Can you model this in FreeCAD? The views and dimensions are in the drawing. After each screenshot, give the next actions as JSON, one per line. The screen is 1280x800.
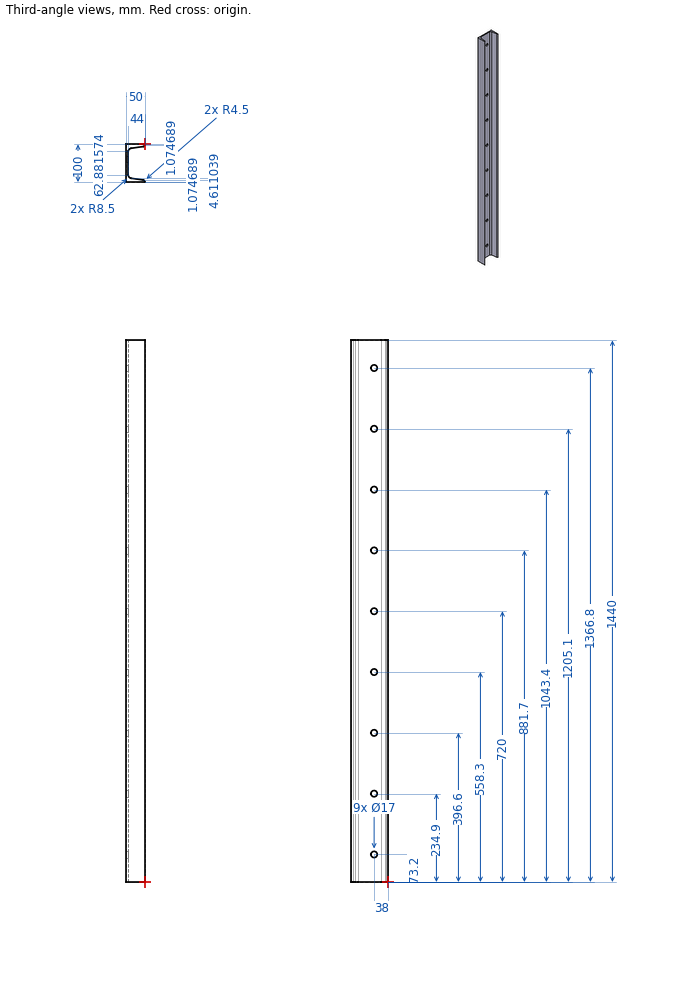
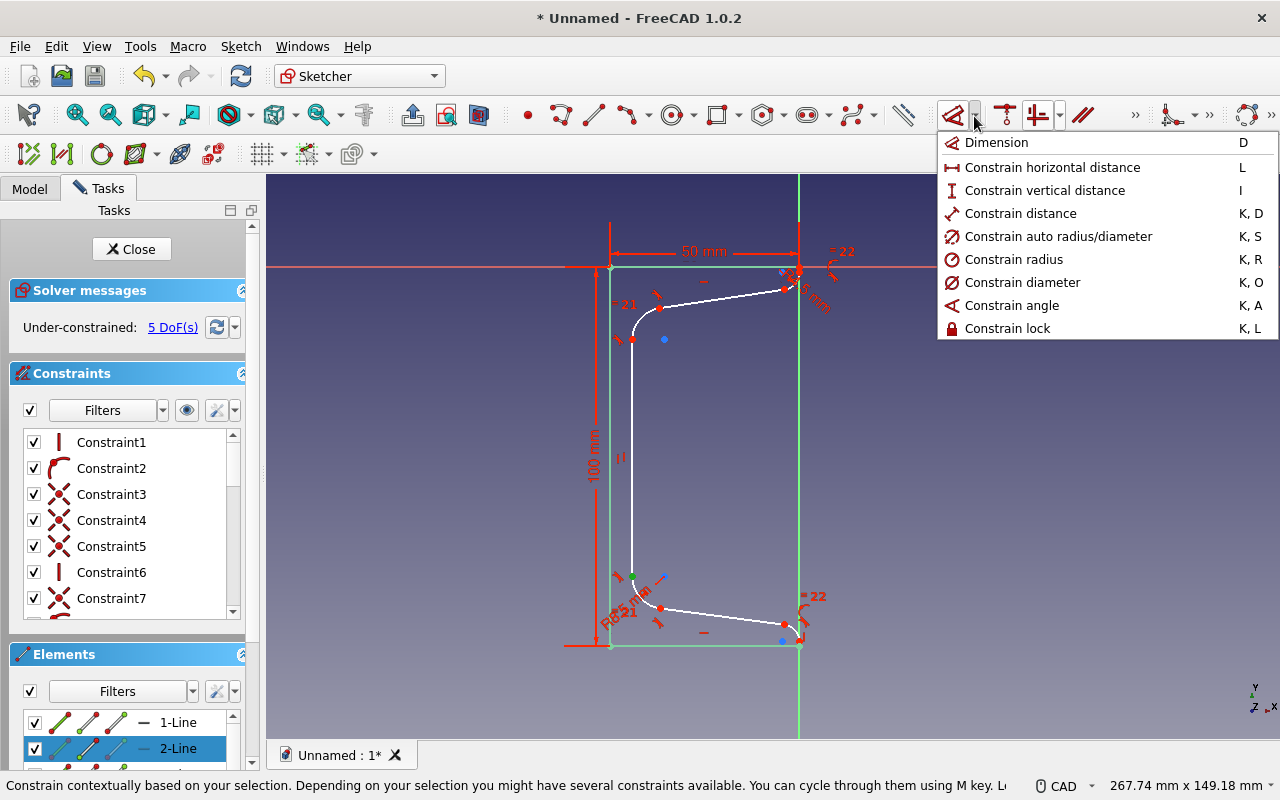
{"action": "left_click", "coordinate": [1108, 168]}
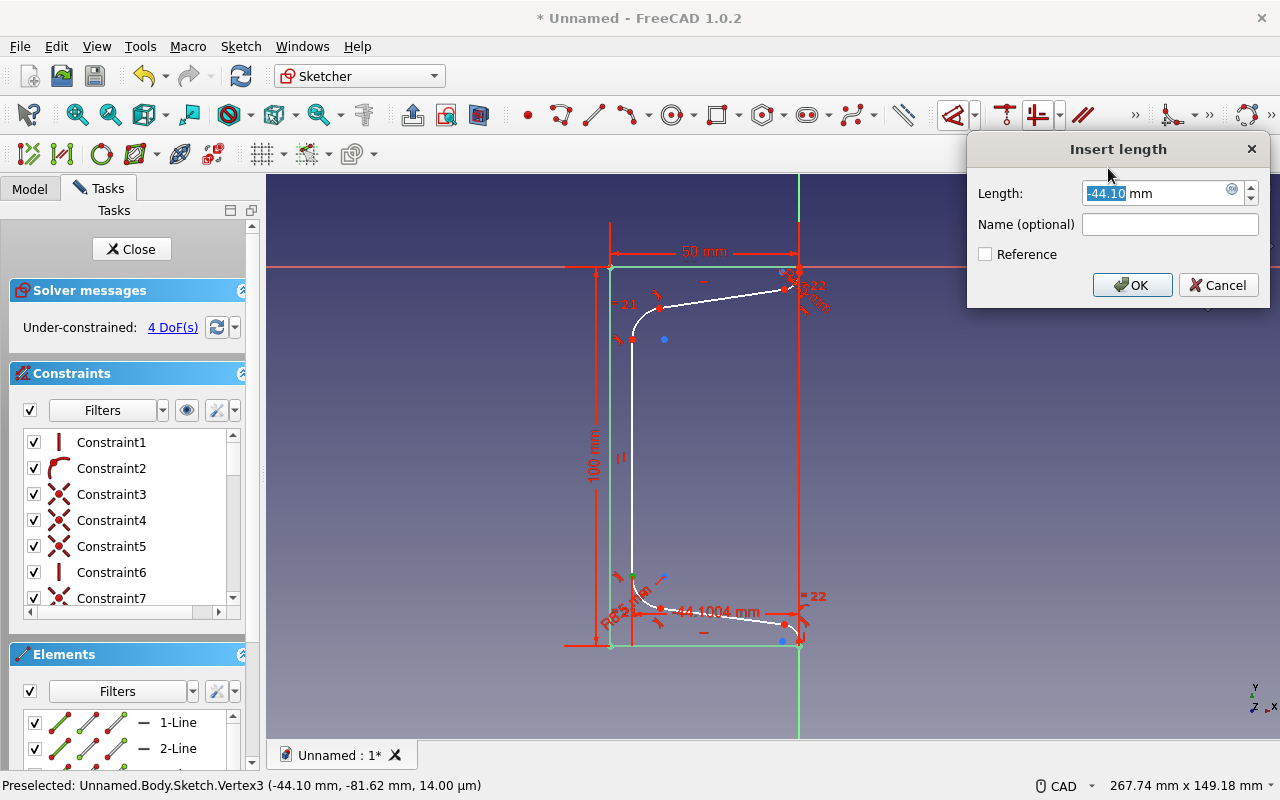
{"action": "type", "text": "-44"}
{"action": "key", "text": "Return"}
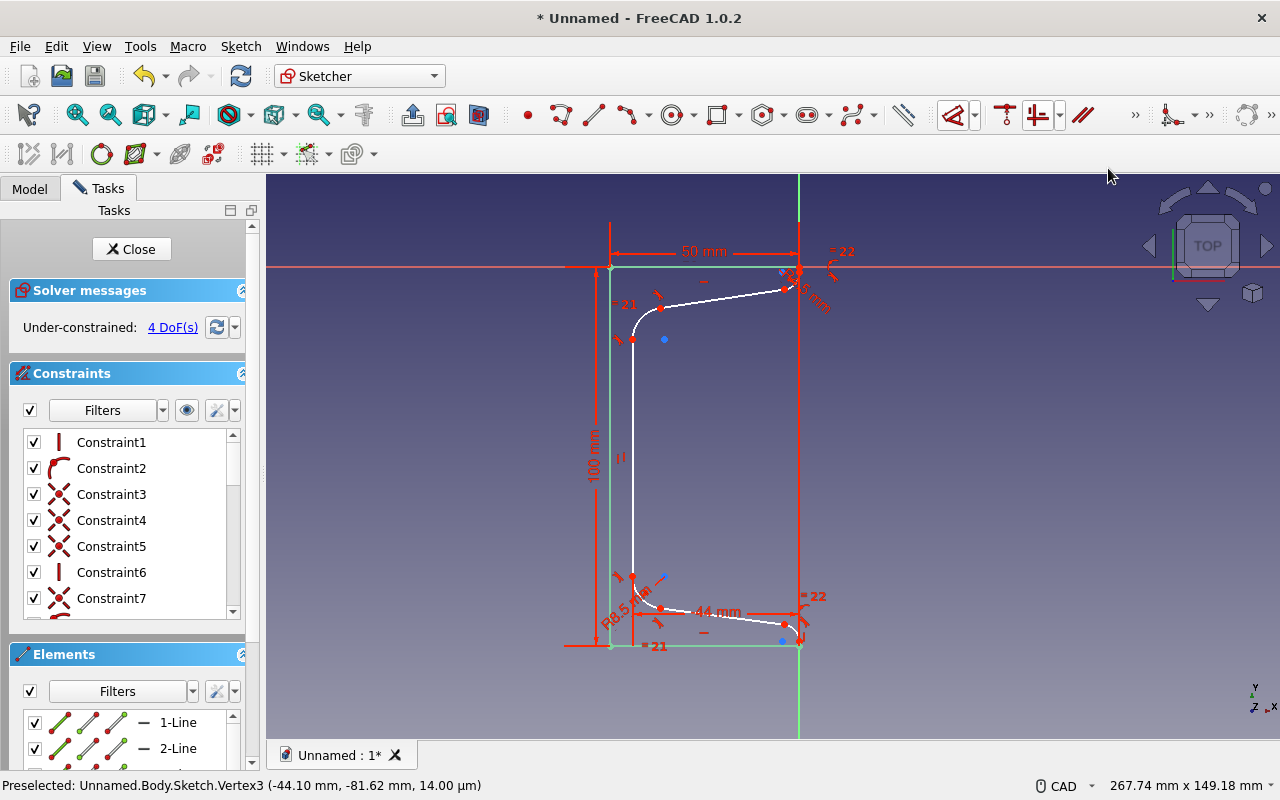
{"action": "scroll", "coordinate": [799, 270], "scroll_direction": "up", "scroll_amount": 12}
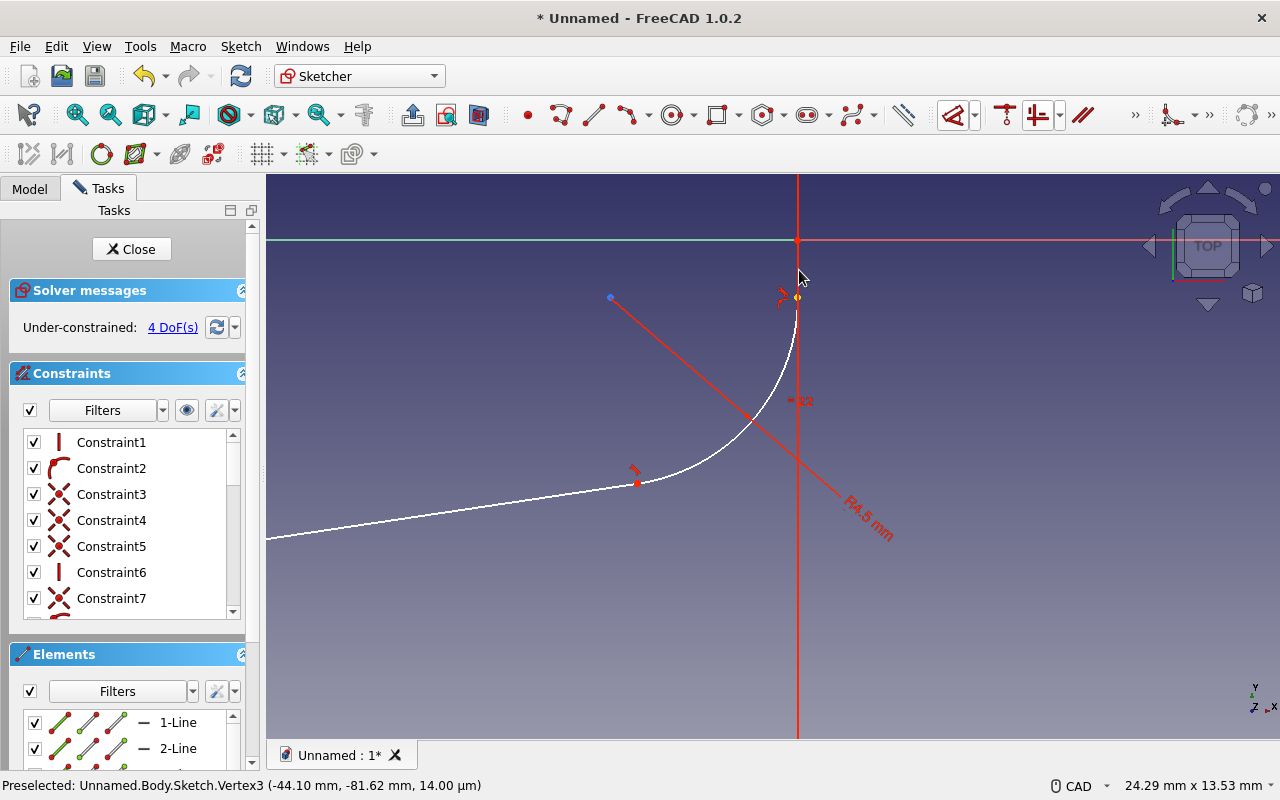
{"action": "left_click", "coordinate": [798, 269]}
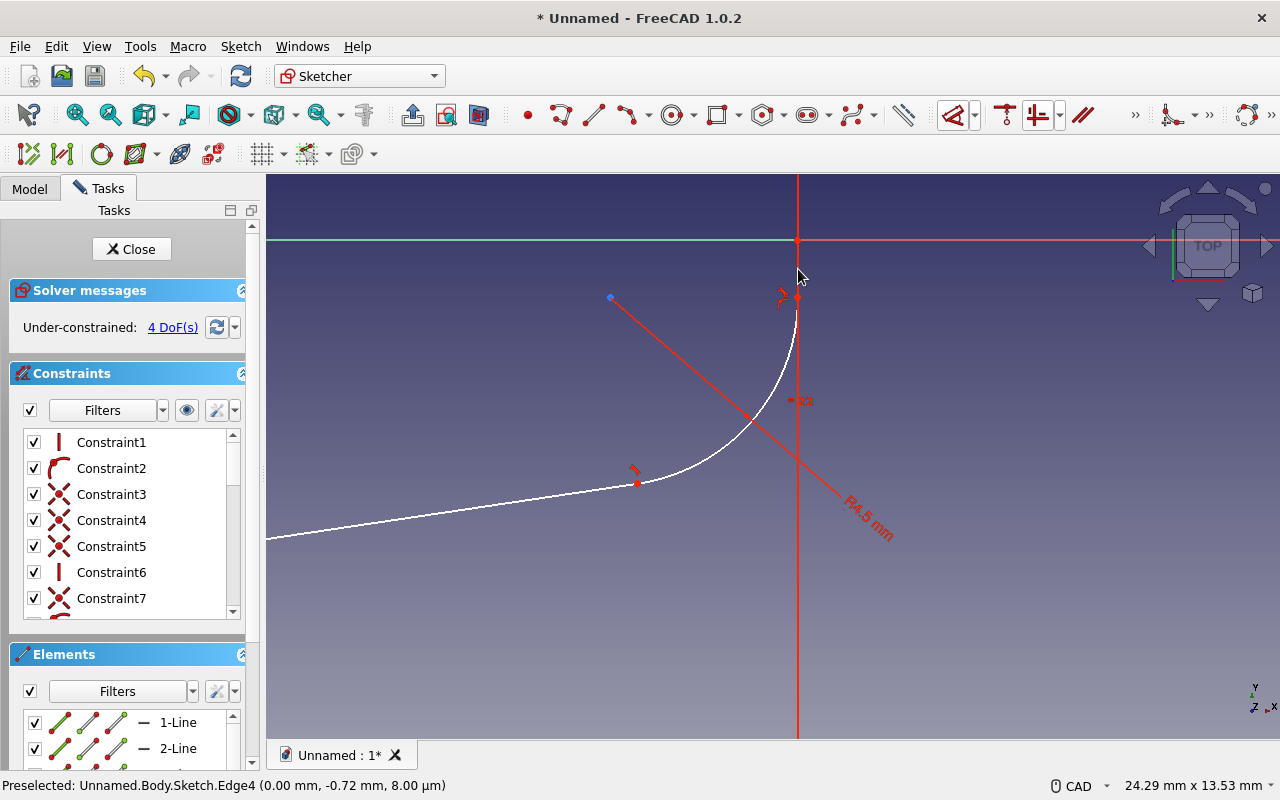
{"action": "left_click", "coordinate": [974, 116]}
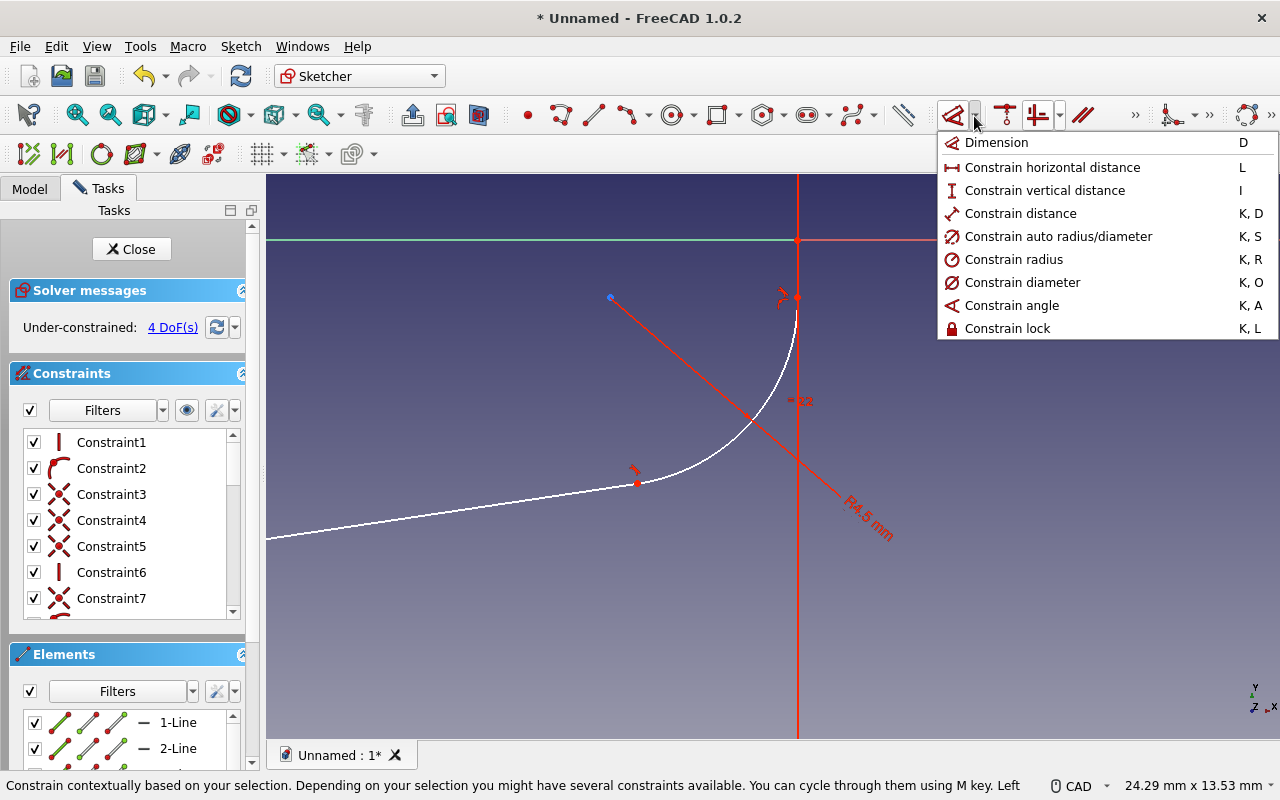
{"action": "left_click", "coordinate": [1108, 190]}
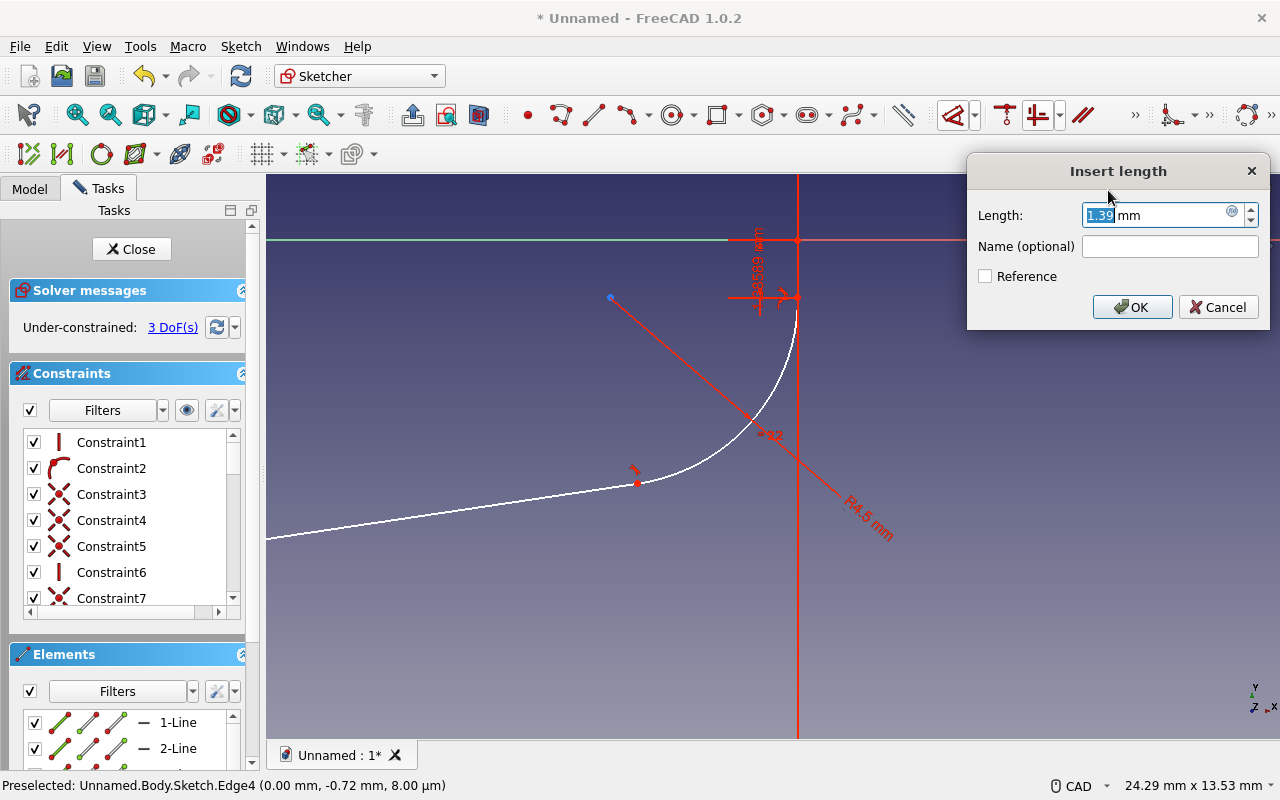
{"action": "type", "text": "1.074689"}
{"action": "key", "text": "Return"}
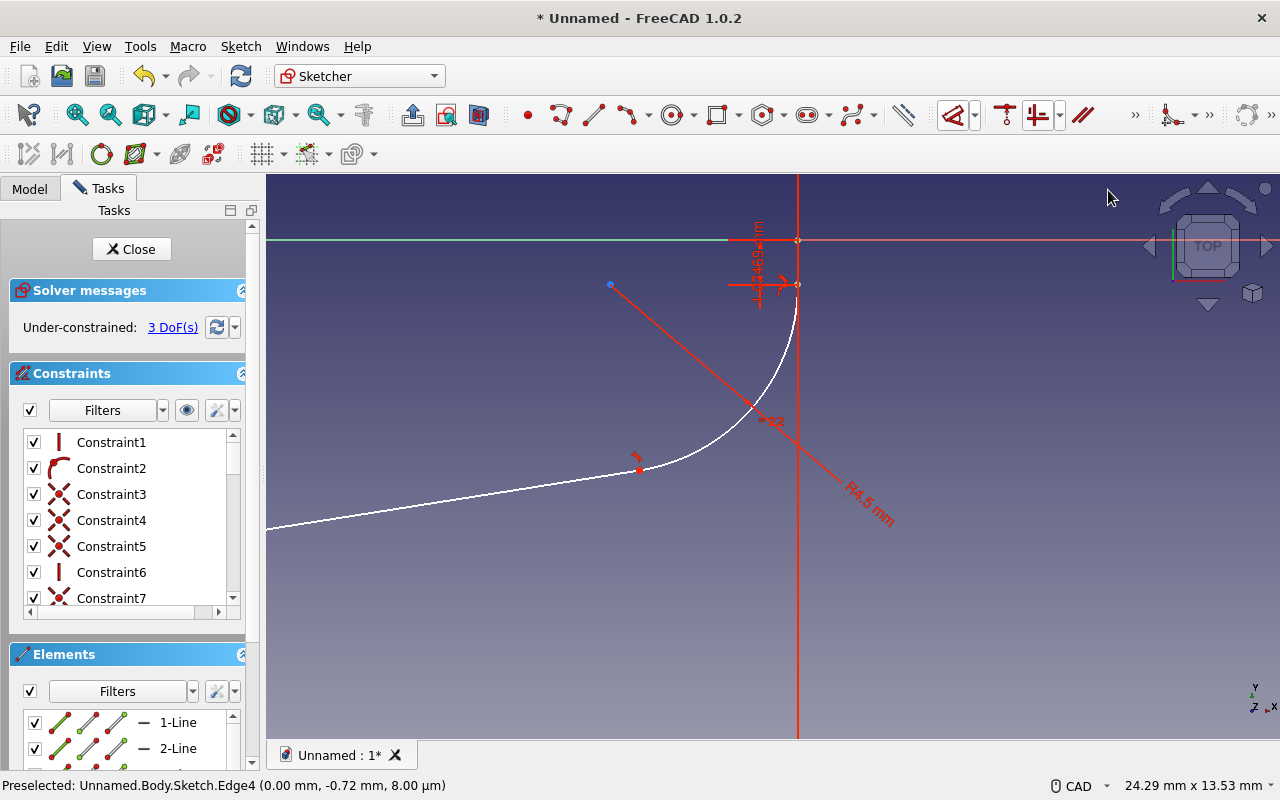
{"action": "scroll", "coordinate": [799, 270], "scroll_direction": "down", "scroll_amount": 12}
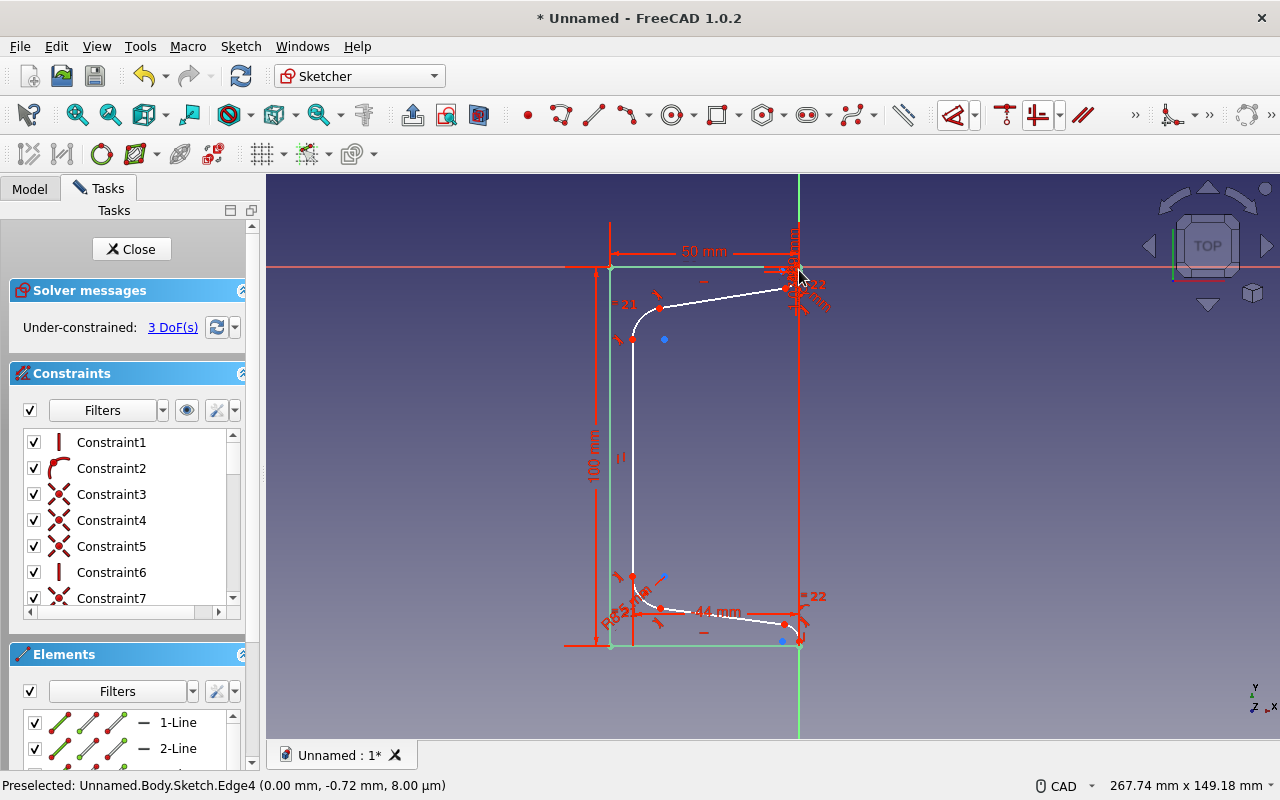
{"action": "scroll", "coordinate": [799, 645], "scroll_direction": "up", "scroll_amount": 12}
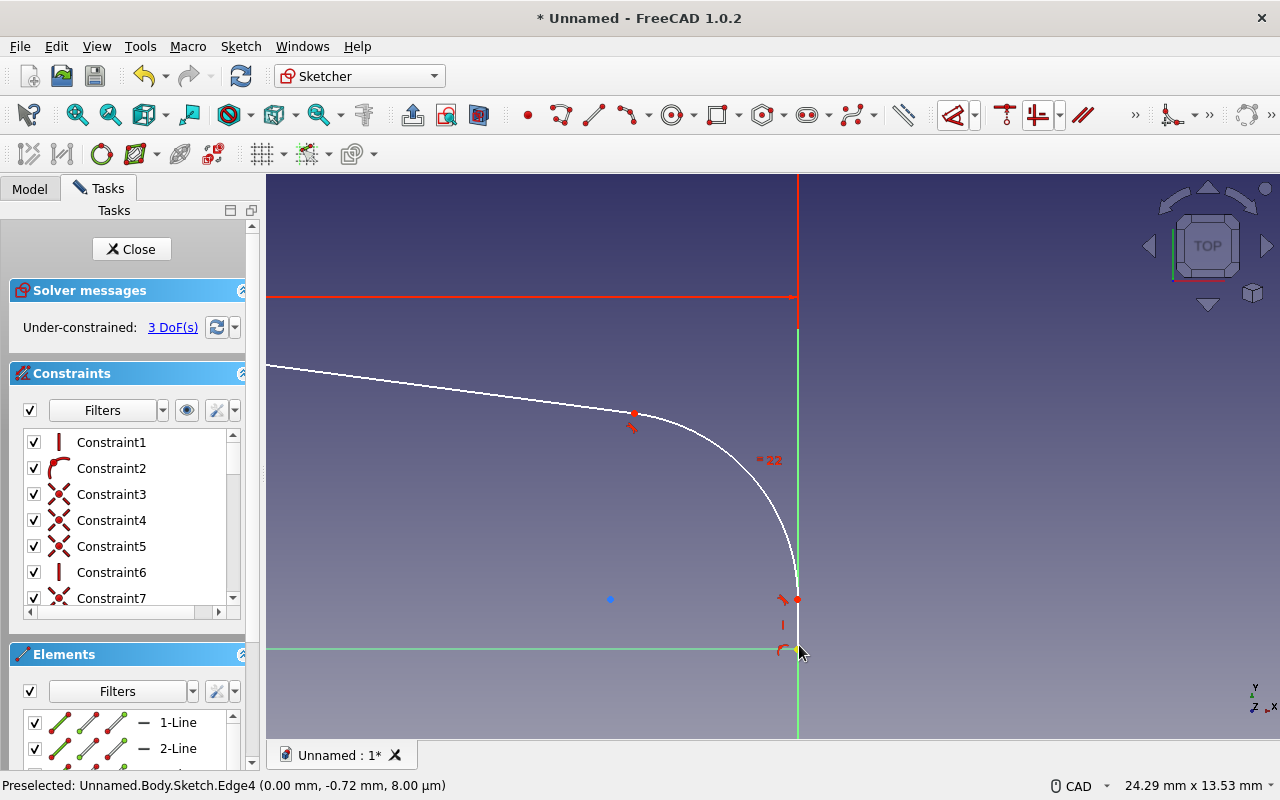
{"action": "left_click", "coordinate": [798, 635]}